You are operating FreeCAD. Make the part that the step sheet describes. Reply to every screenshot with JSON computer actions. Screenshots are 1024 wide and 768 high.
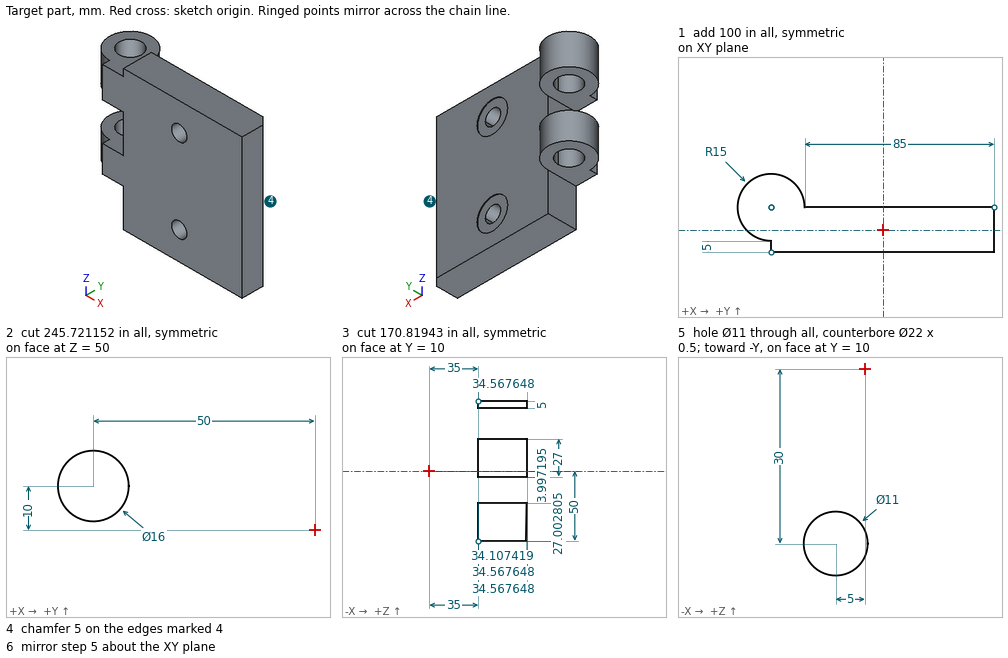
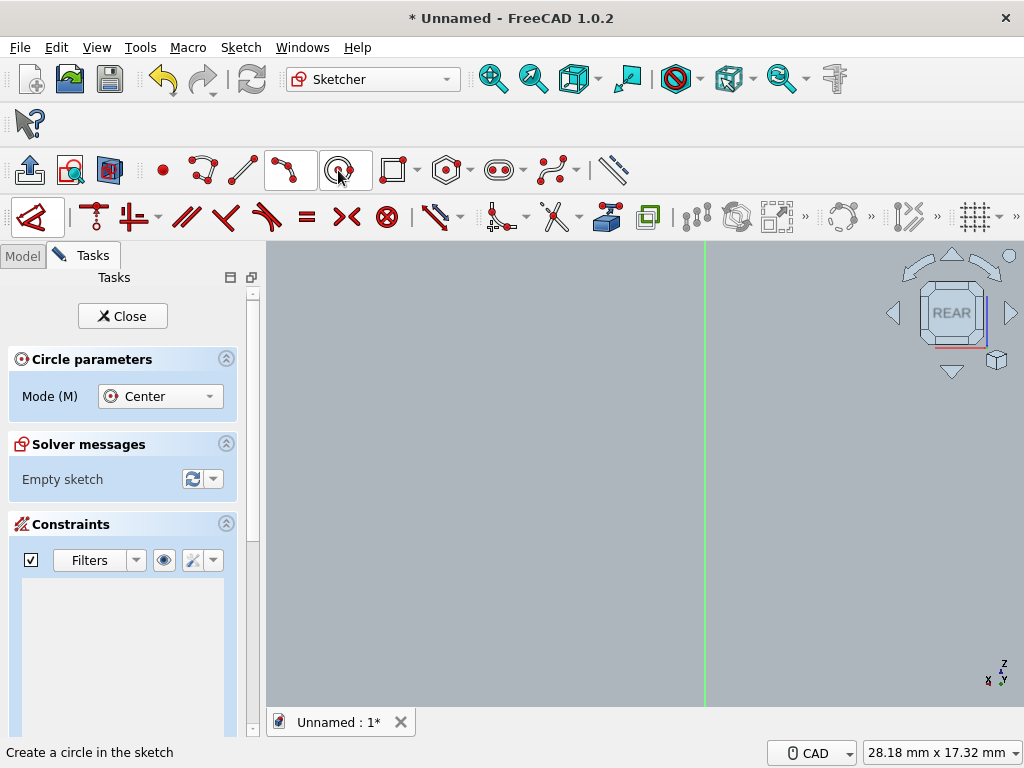
{"action": "left_click", "coordinate": [570, 465]}
{"action": "mouse_move", "coordinate": [675, 360]}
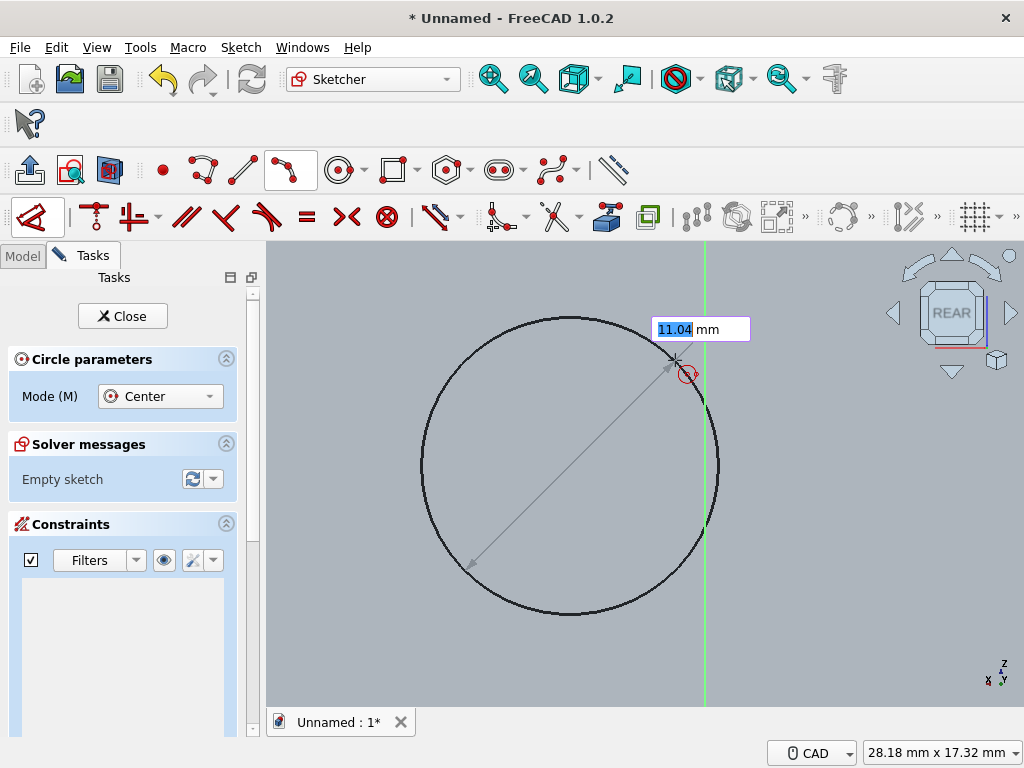
{"action": "type", "text": "11"}
{"action": "key", "text": "Return"}
{"action": "key", "text": "Escape"}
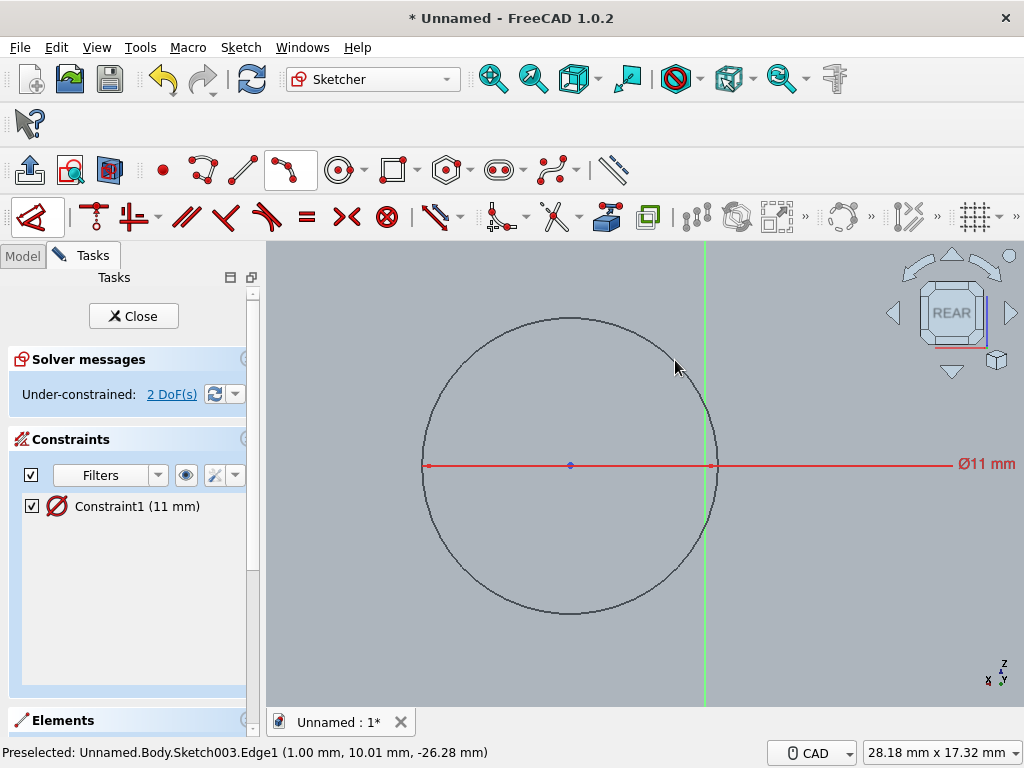
{"action": "left_click", "coordinate": [570, 466]}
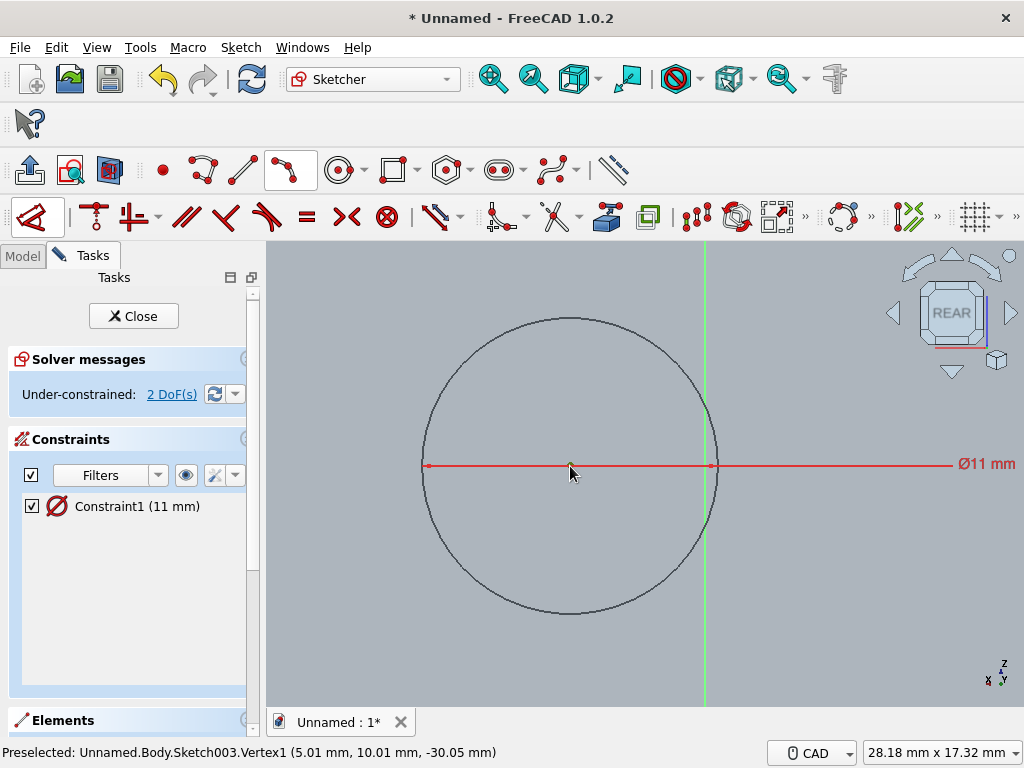
{"action": "key", "text": "l"}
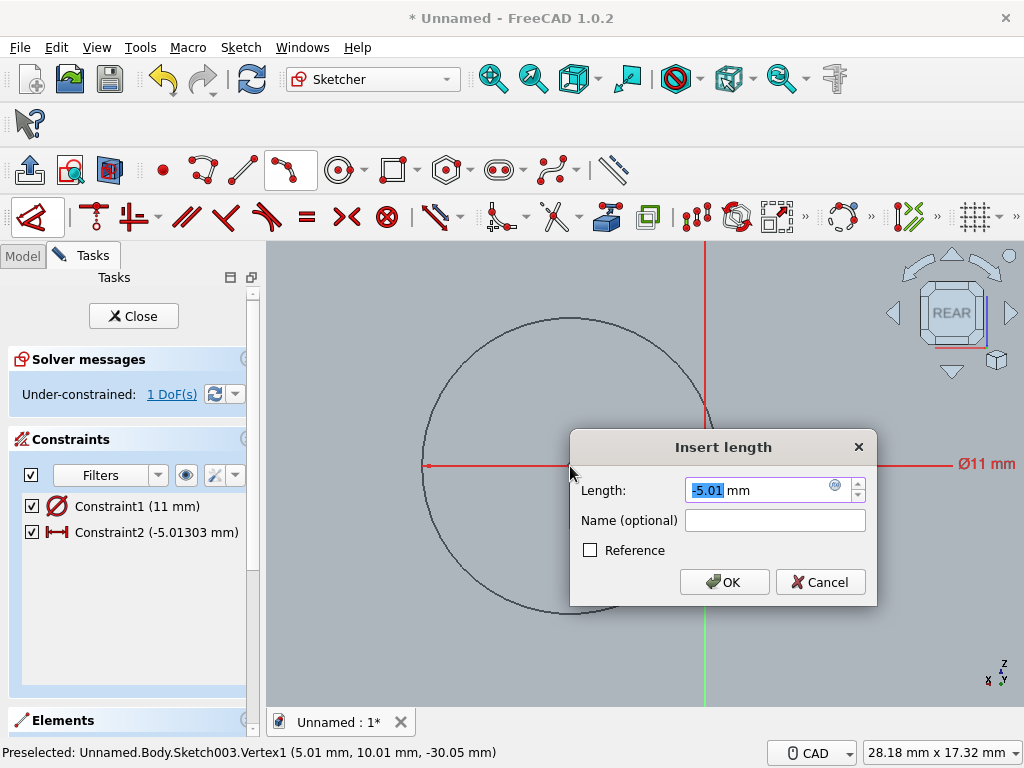
{"action": "type", "text": "-5"}
{"action": "key", "text": "Return"}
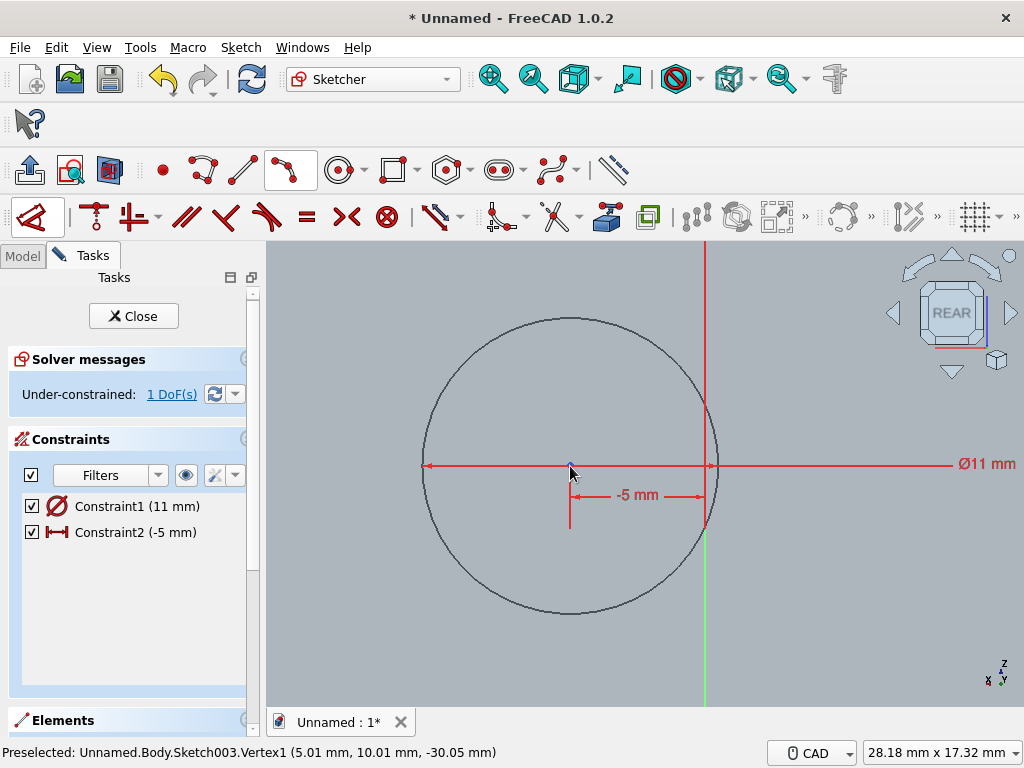
{"action": "left_click", "coordinate": [570, 466]}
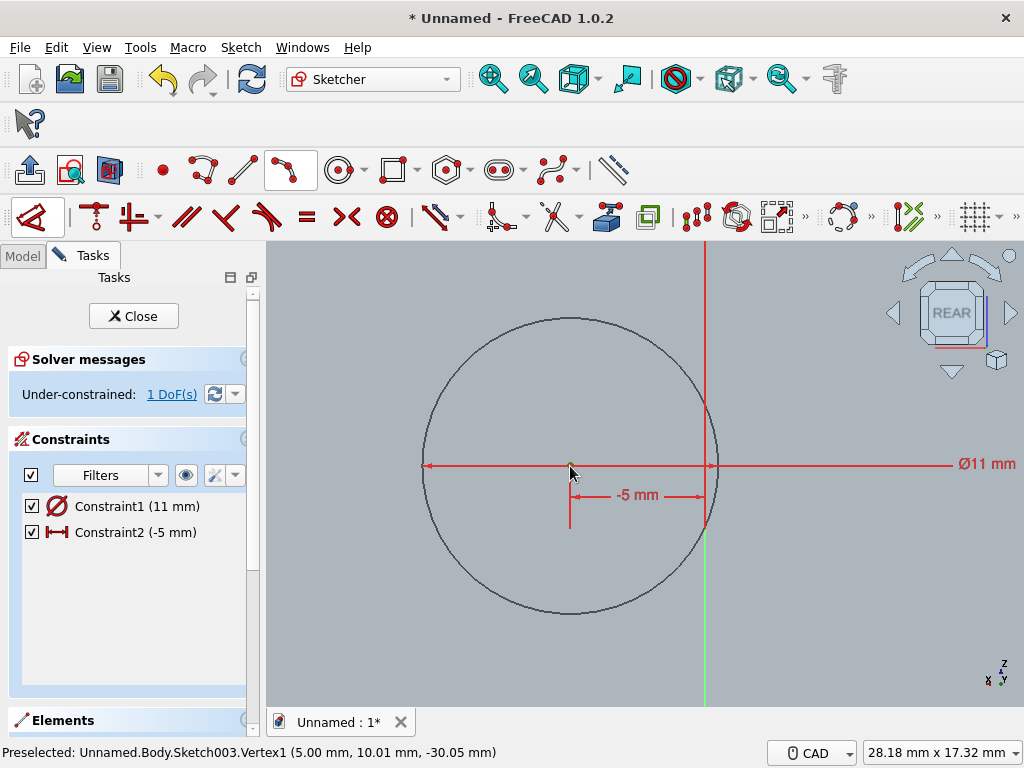
{"action": "left_click", "coordinate": [58, 218]}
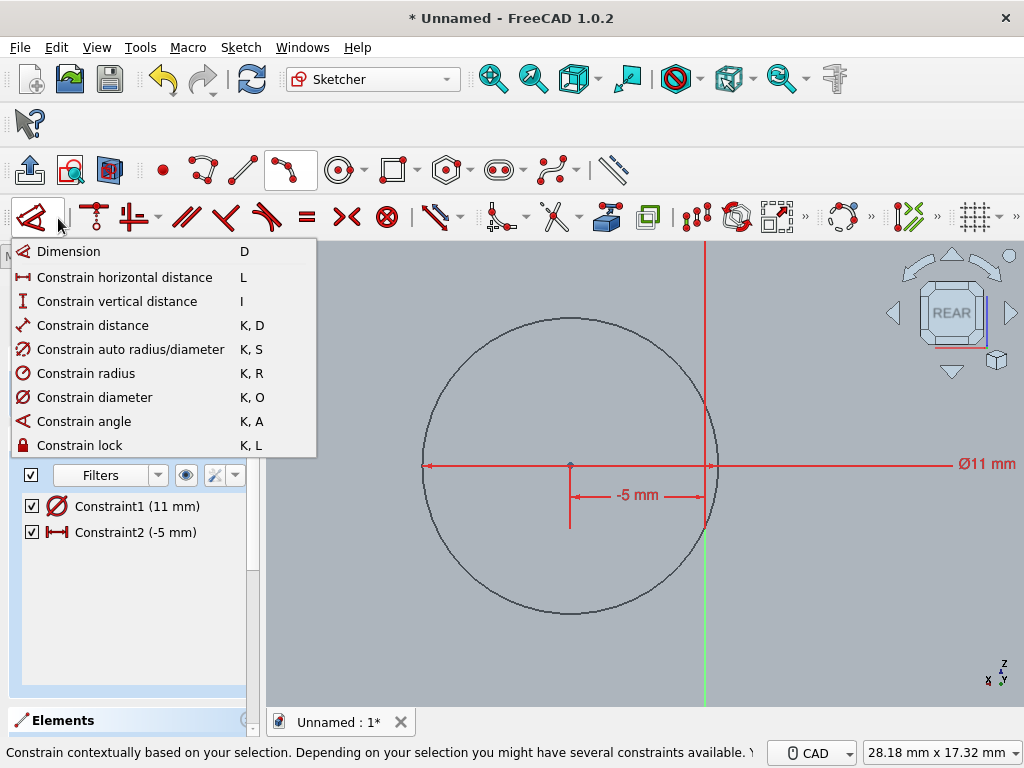
{"action": "left_click", "coordinate": [164, 301]}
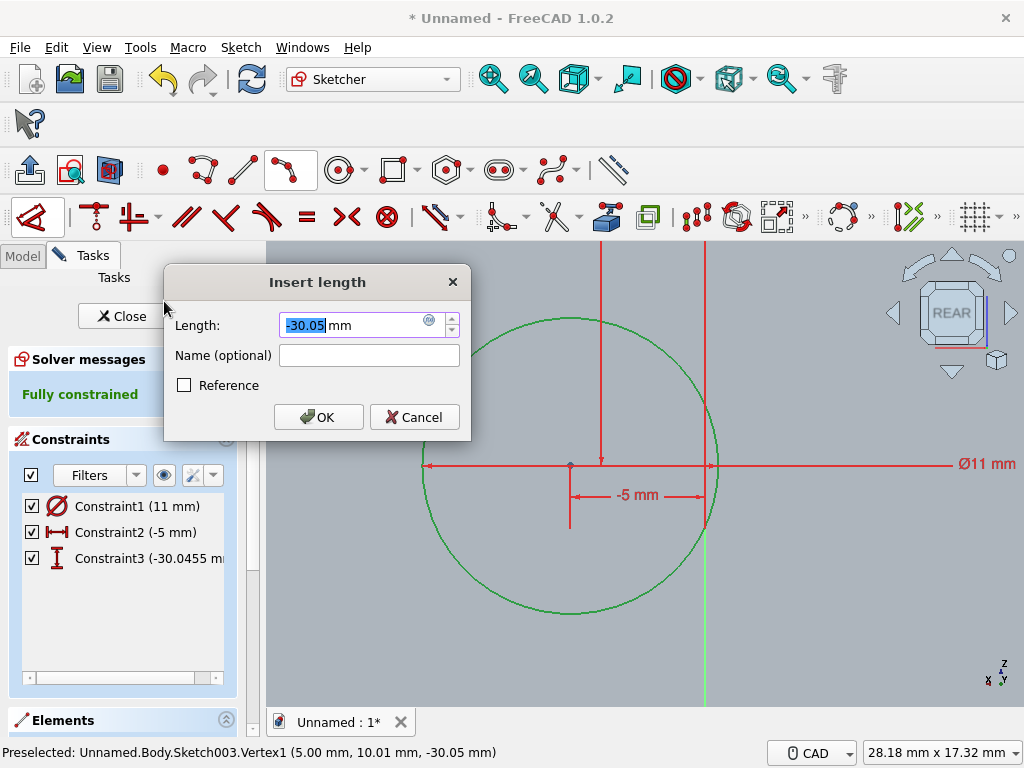
{"action": "type", "text": "-30"}
{"action": "key", "text": "Return"}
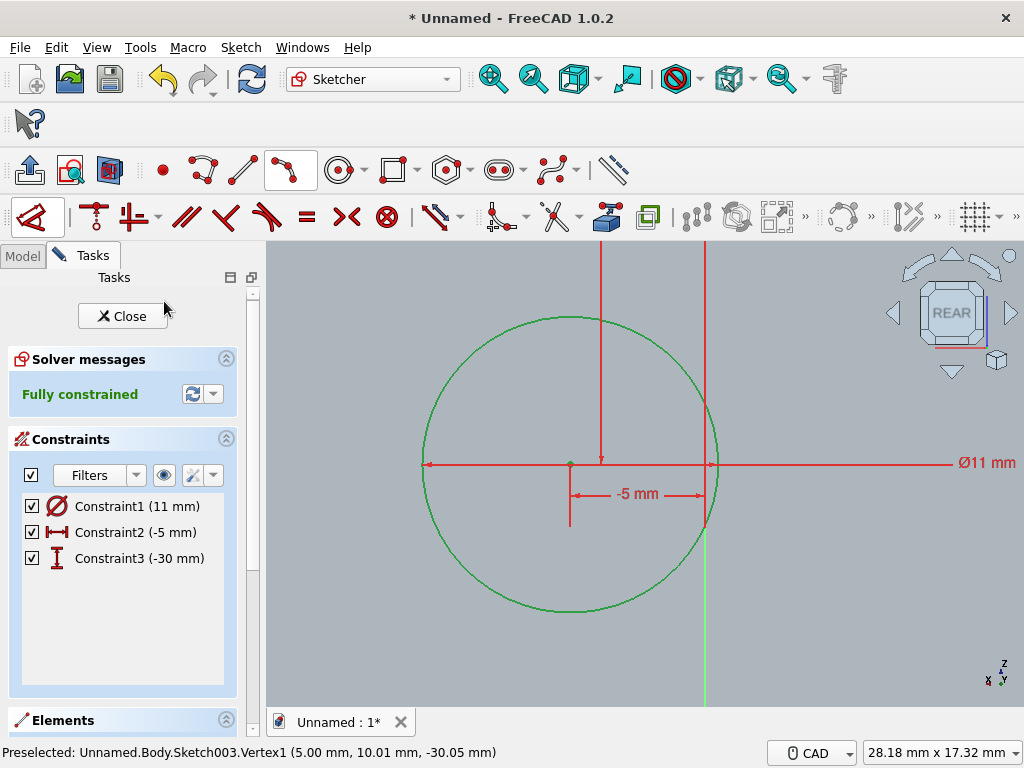
{"action": "left_click", "coordinate": [123, 316]}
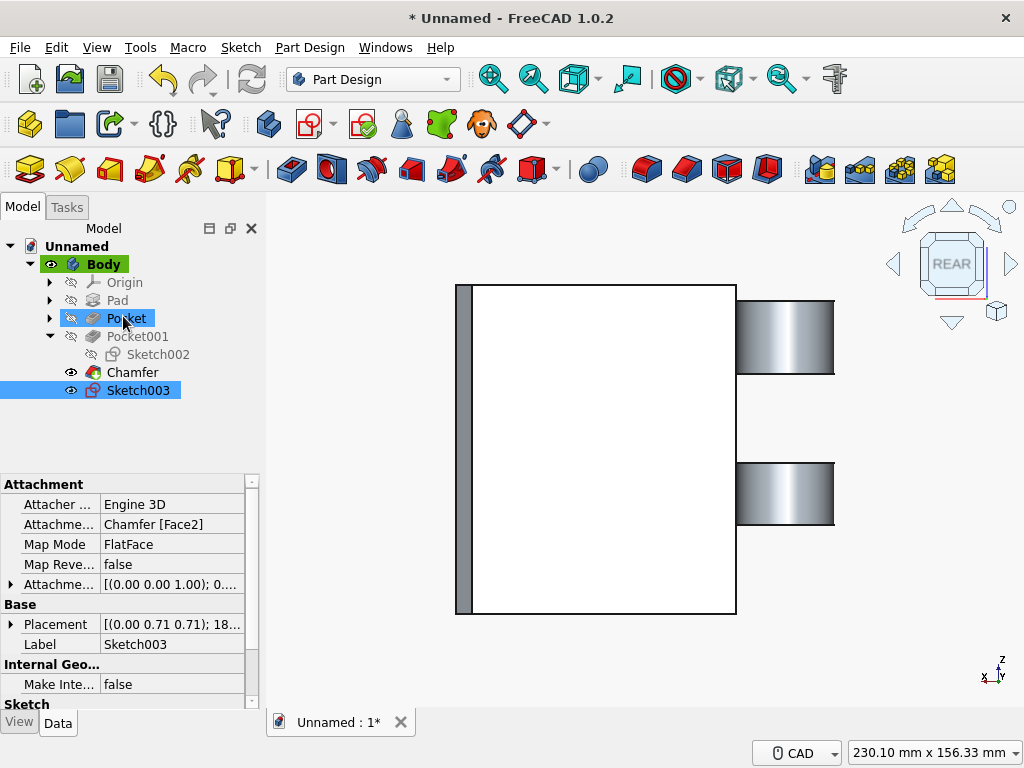
{"action": "left_click", "coordinate": [332, 170]}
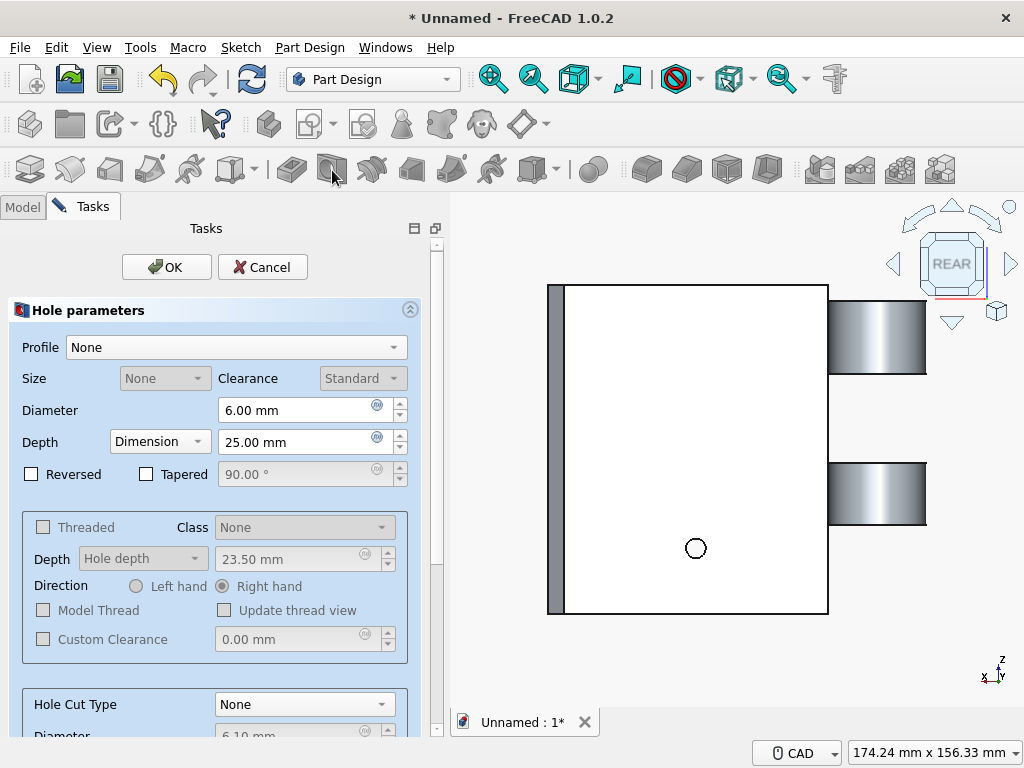
{"action": "triple_click", "coordinate": [305, 410]}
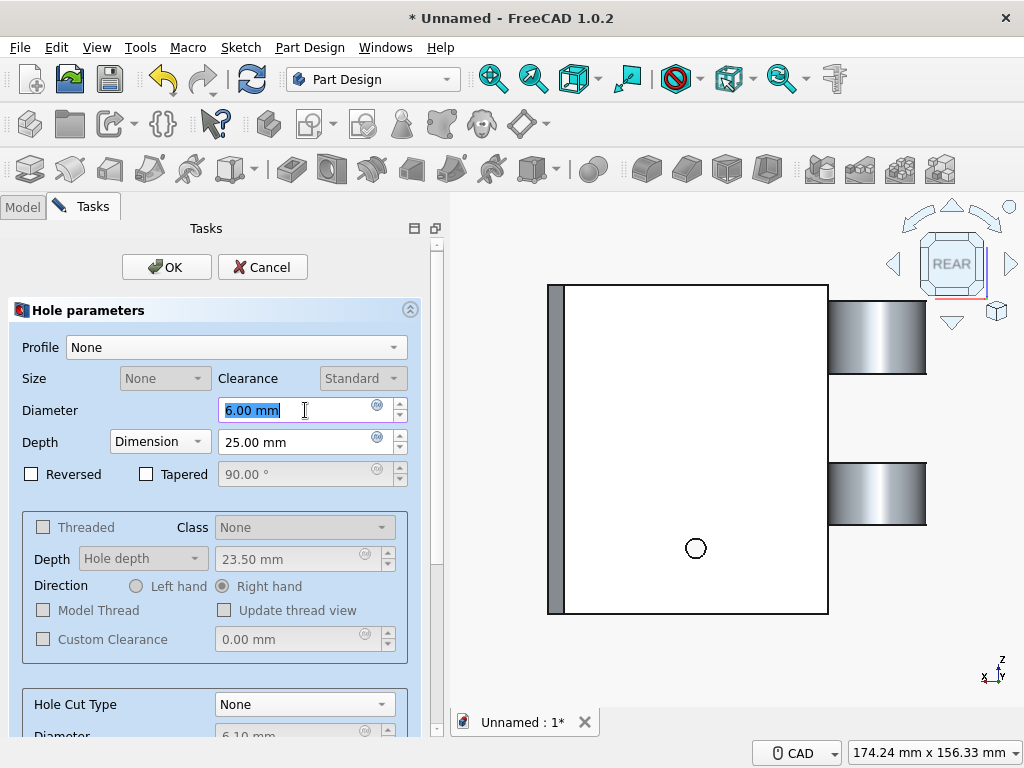
{"action": "type", "text": "11"}
{"action": "key", "text": "Tab"}